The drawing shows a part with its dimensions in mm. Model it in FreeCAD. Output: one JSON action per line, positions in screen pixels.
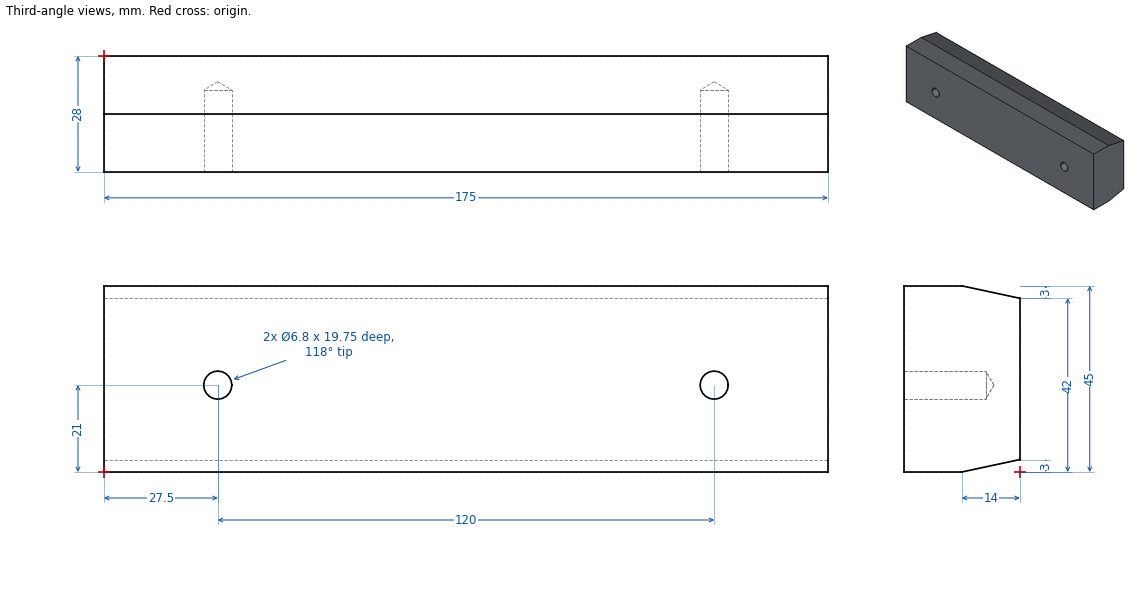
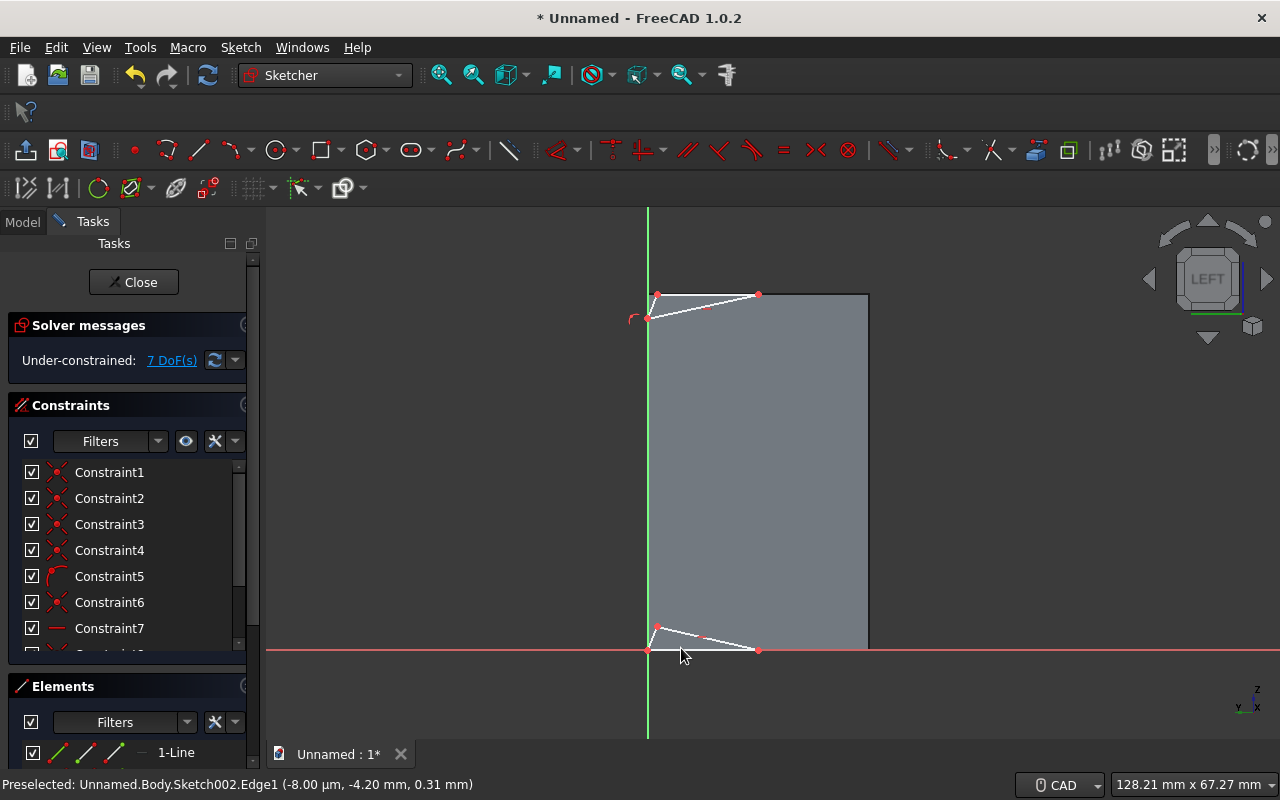
{"action": "scroll", "coordinate": [651, 641], "scroll_direction": "up", "scroll_amount": 3}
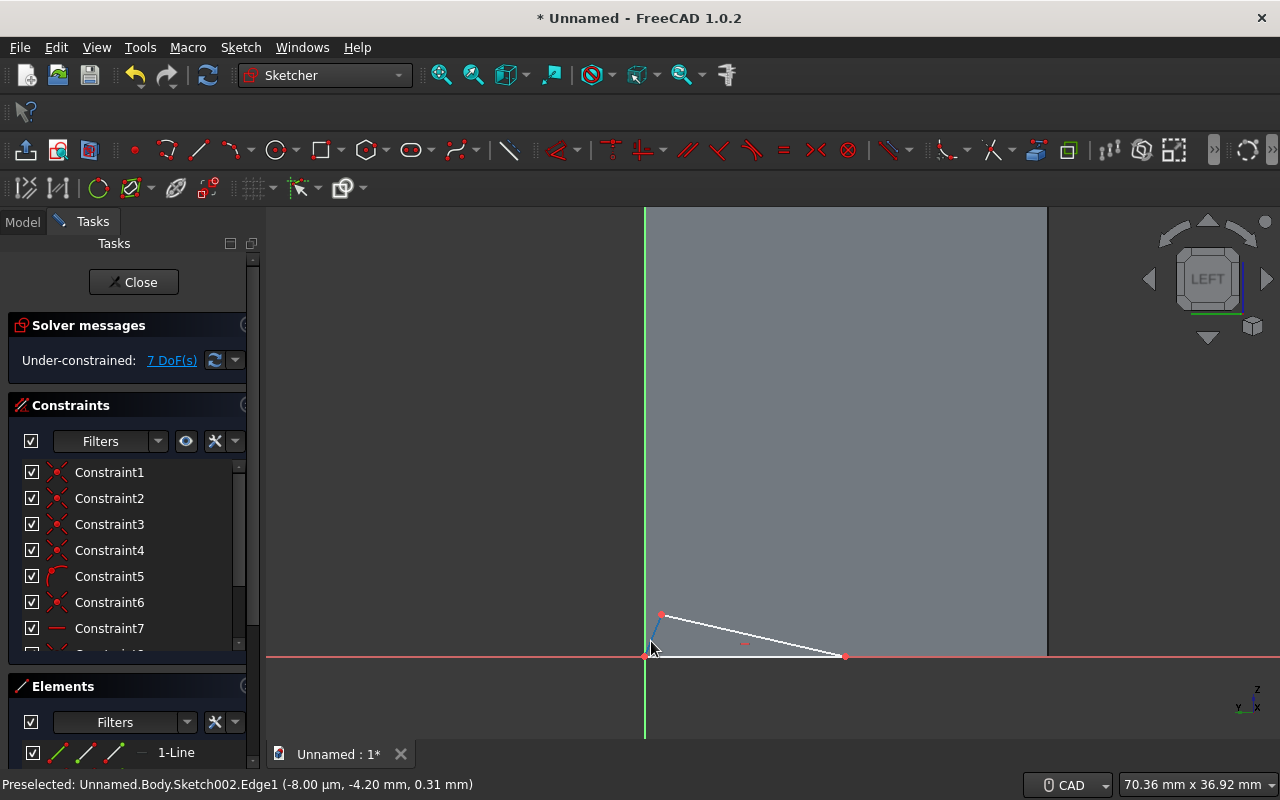
{"action": "left_click", "coordinate": [651, 640]}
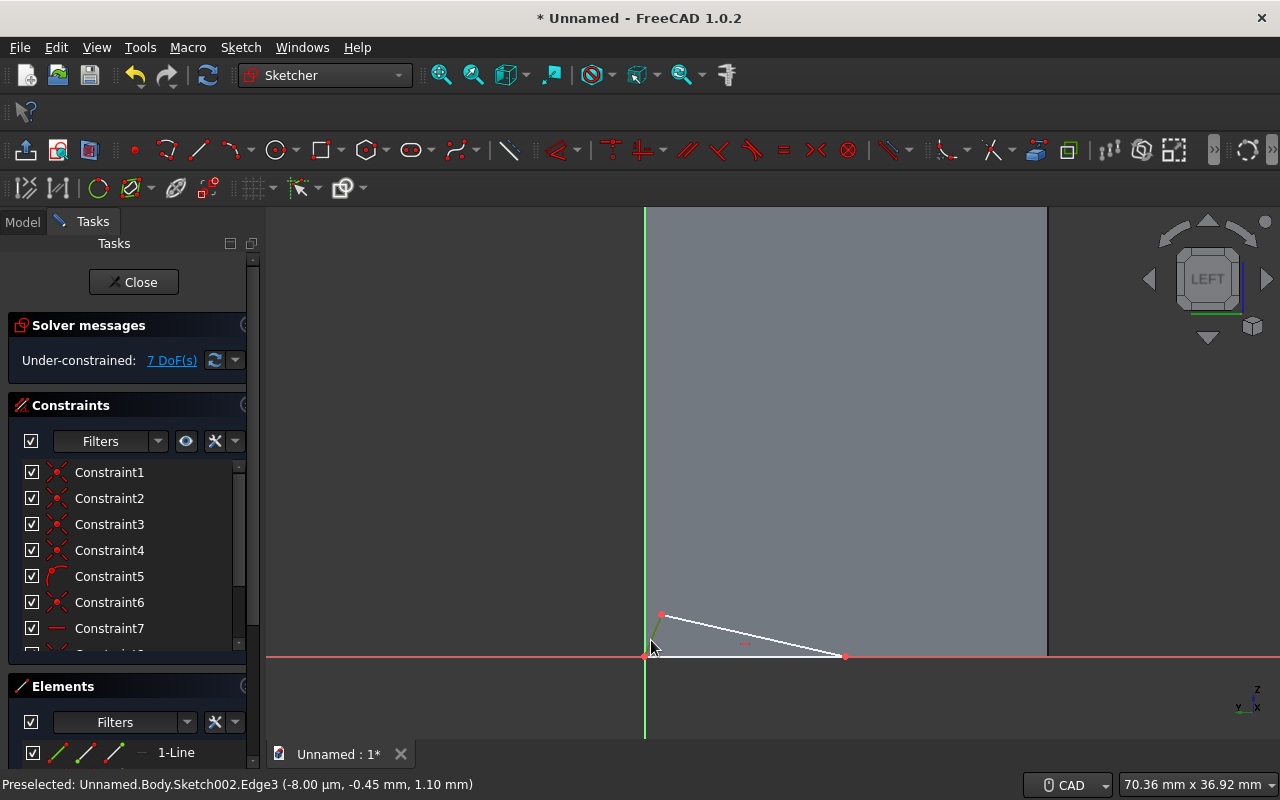
{"action": "key", "text": "v"}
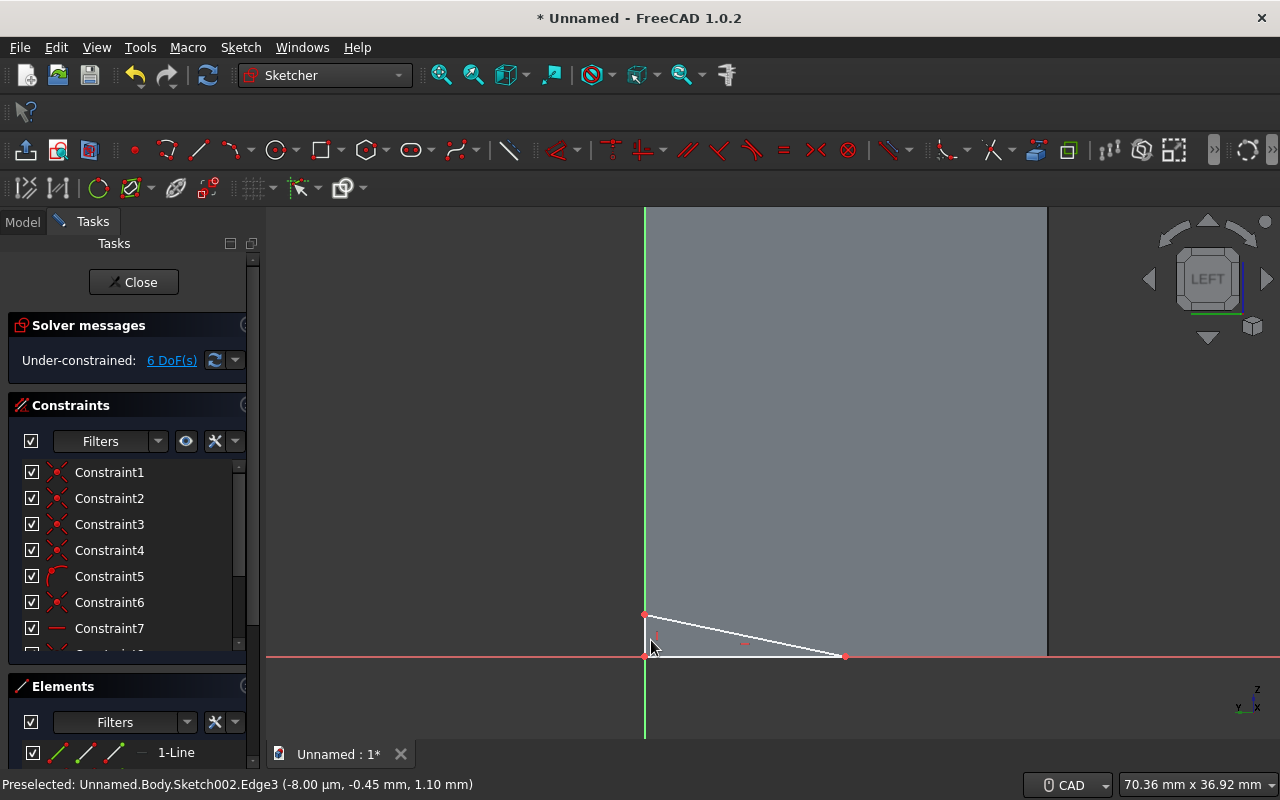
{"action": "scroll", "coordinate": [655, 644], "scroll_direction": "down", "scroll_amount": 3}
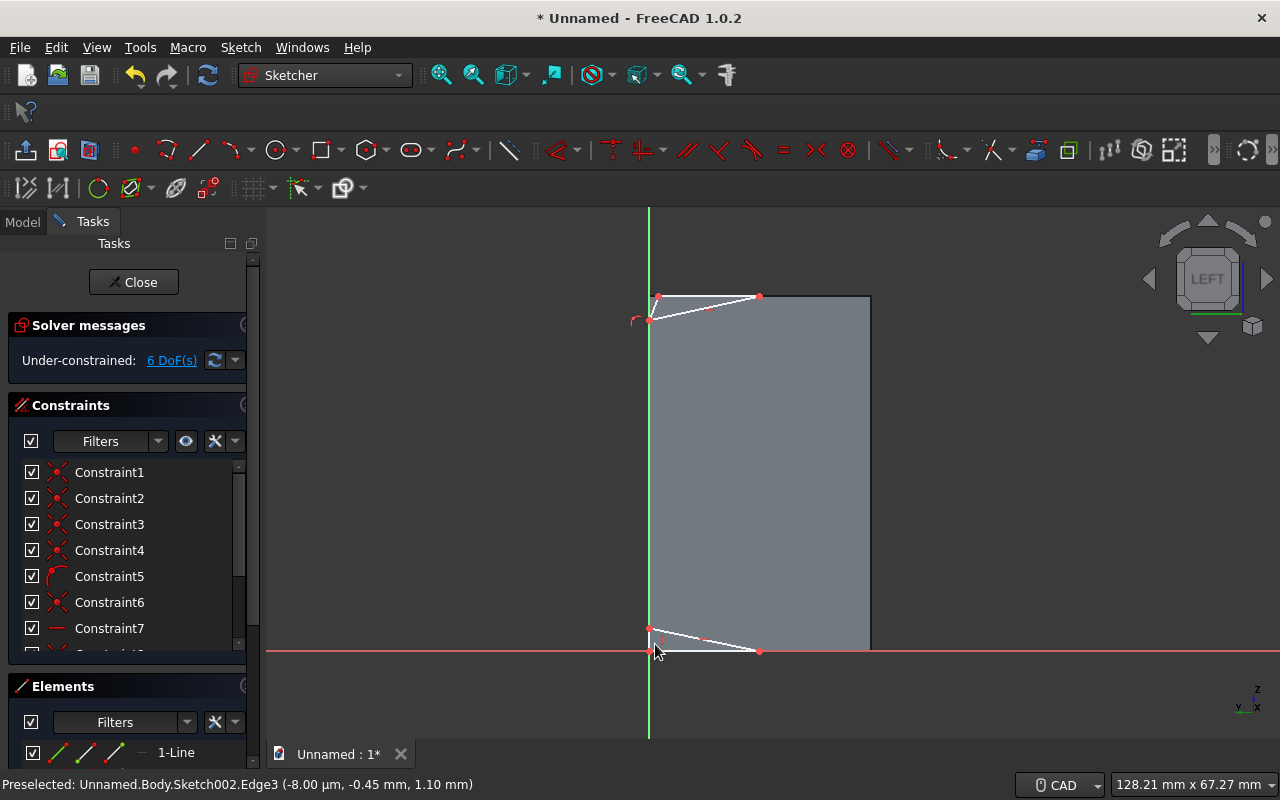
{"action": "scroll", "coordinate": [656, 304], "scroll_direction": "up", "scroll_amount": 4}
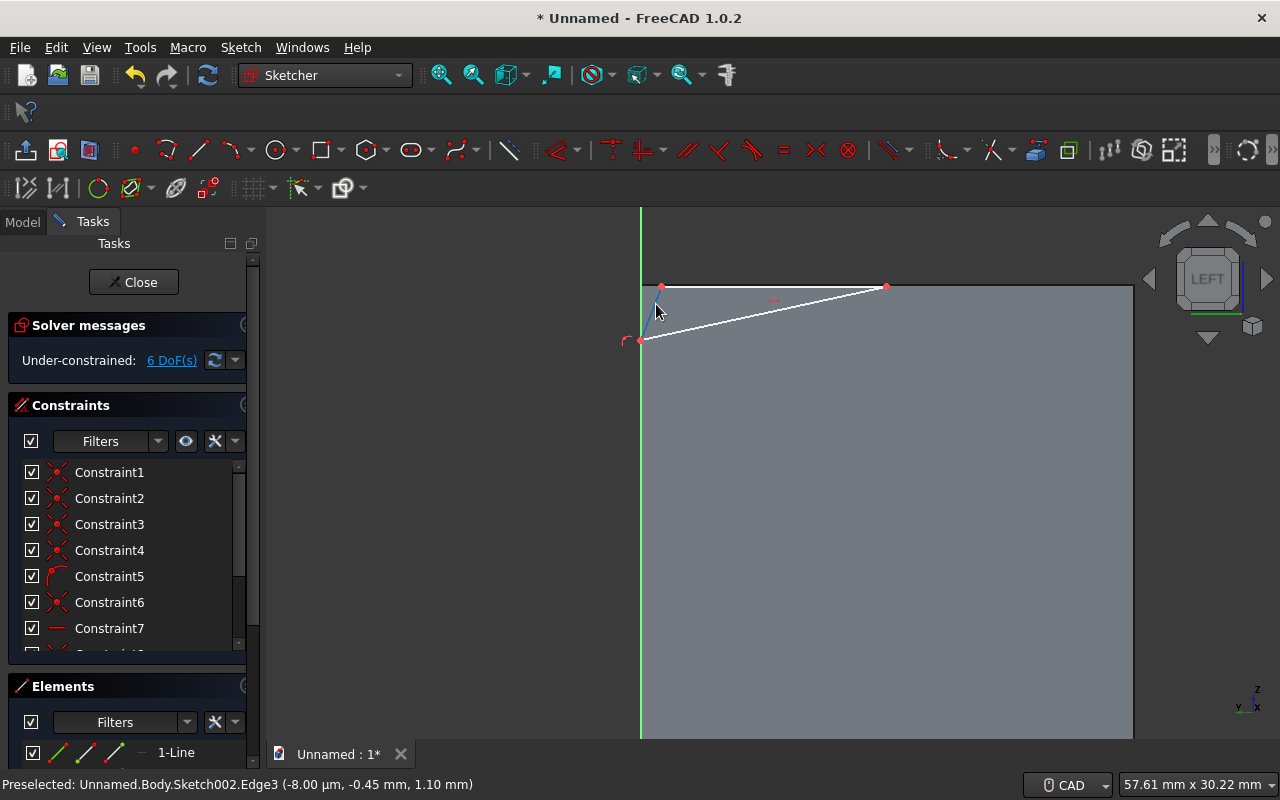
{"action": "left_click", "coordinate": [656, 303]}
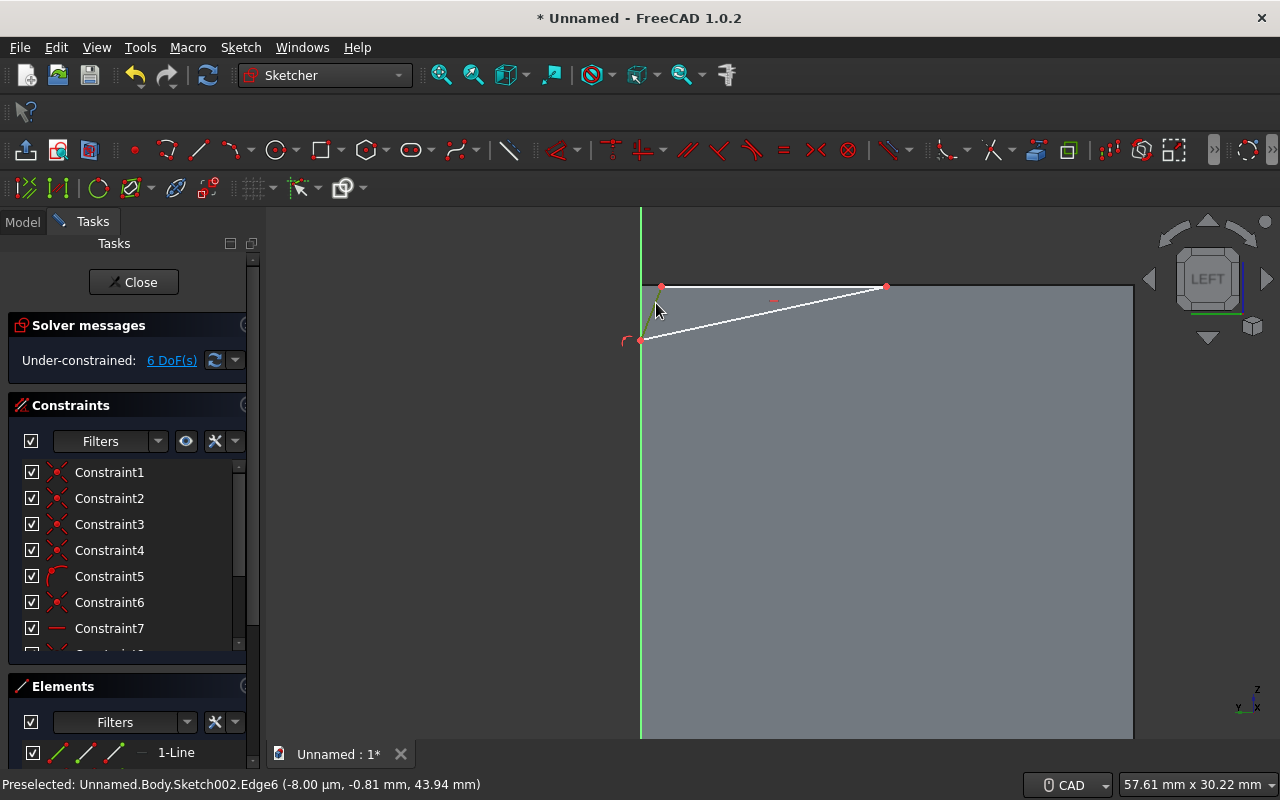
{"action": "key", "text": "v"}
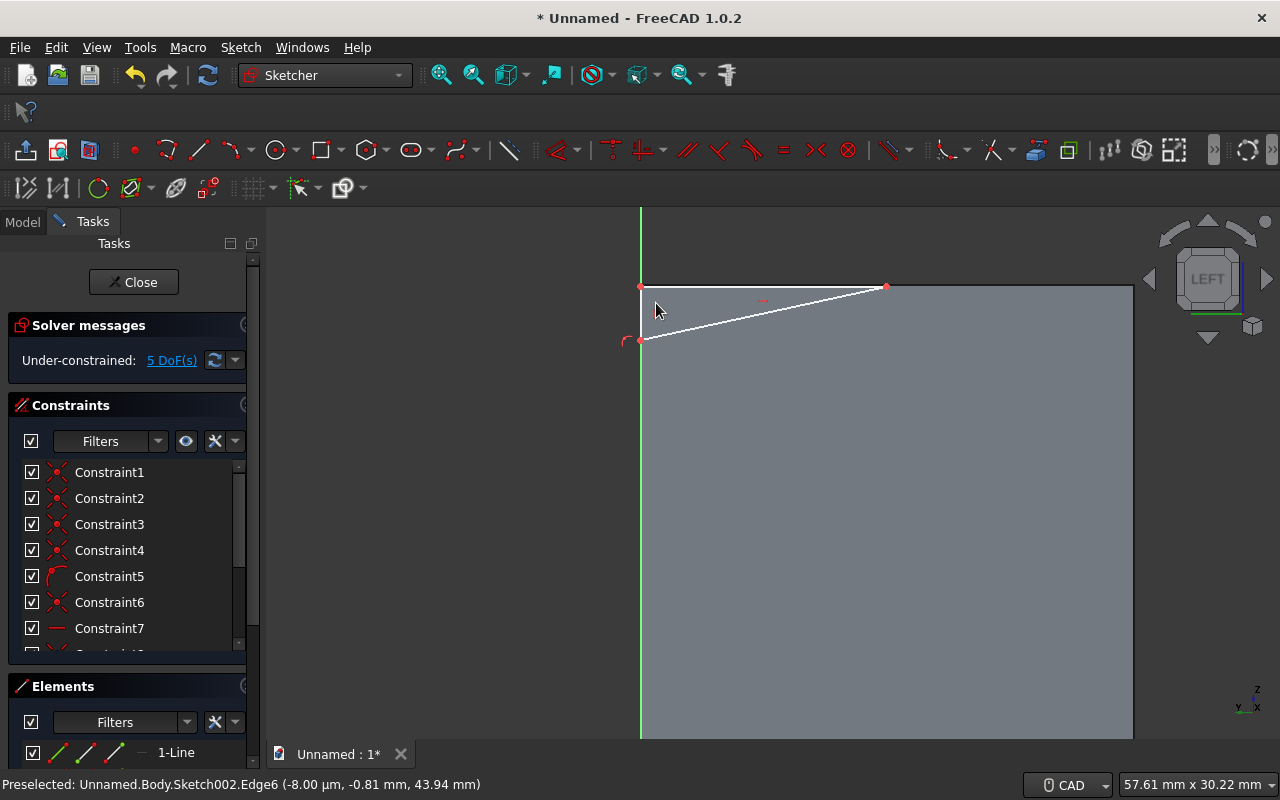
{"action": "key", "text": "d"}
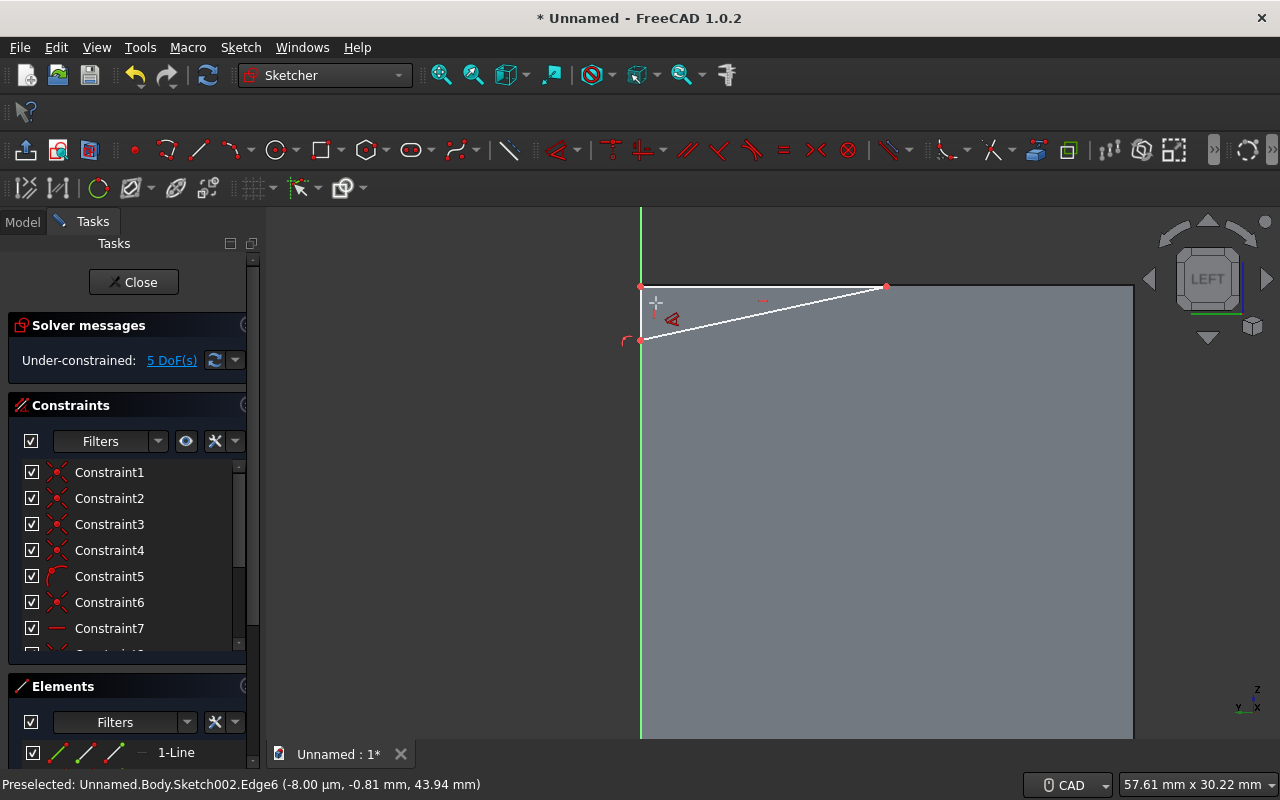
{"action": "scroll", "coordinate": [656, 303], "scroll_direction": "down", "scroll_amount": 4}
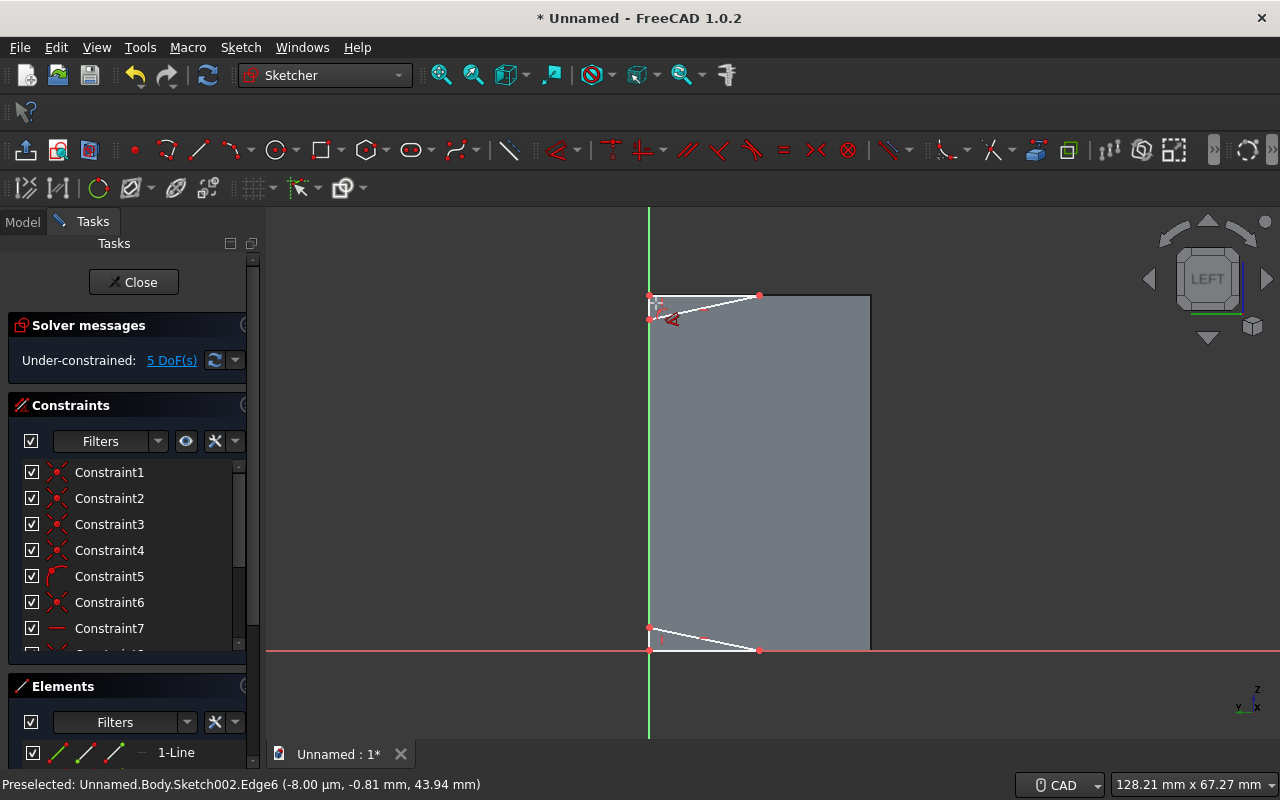
{"action": "scroll", "coordinate": [649, 635], "scroll_direction": "up", "scroll_amount": 4}